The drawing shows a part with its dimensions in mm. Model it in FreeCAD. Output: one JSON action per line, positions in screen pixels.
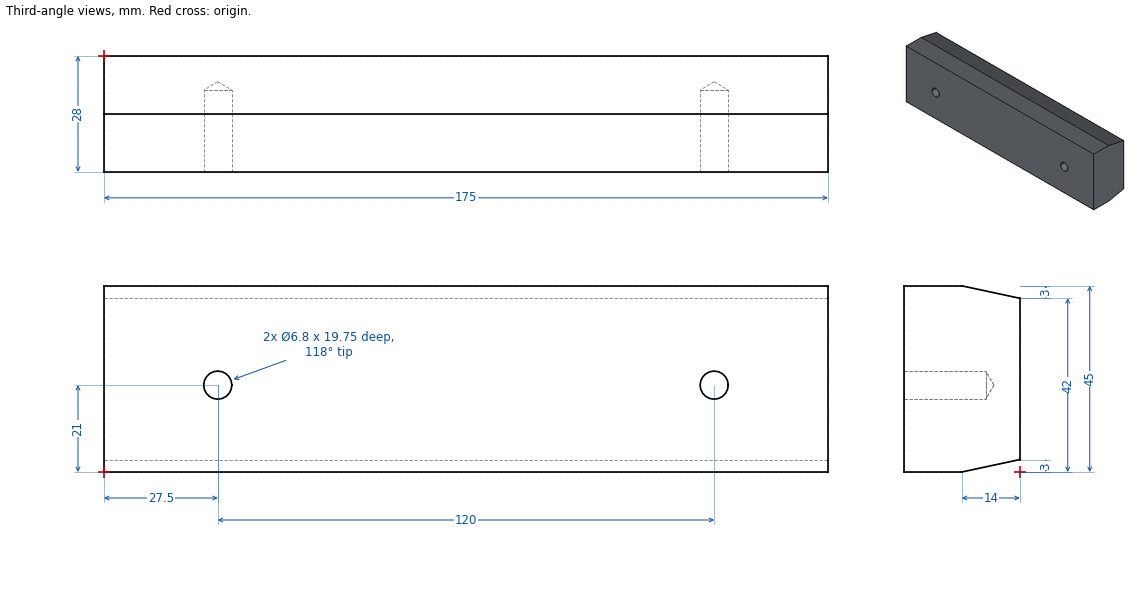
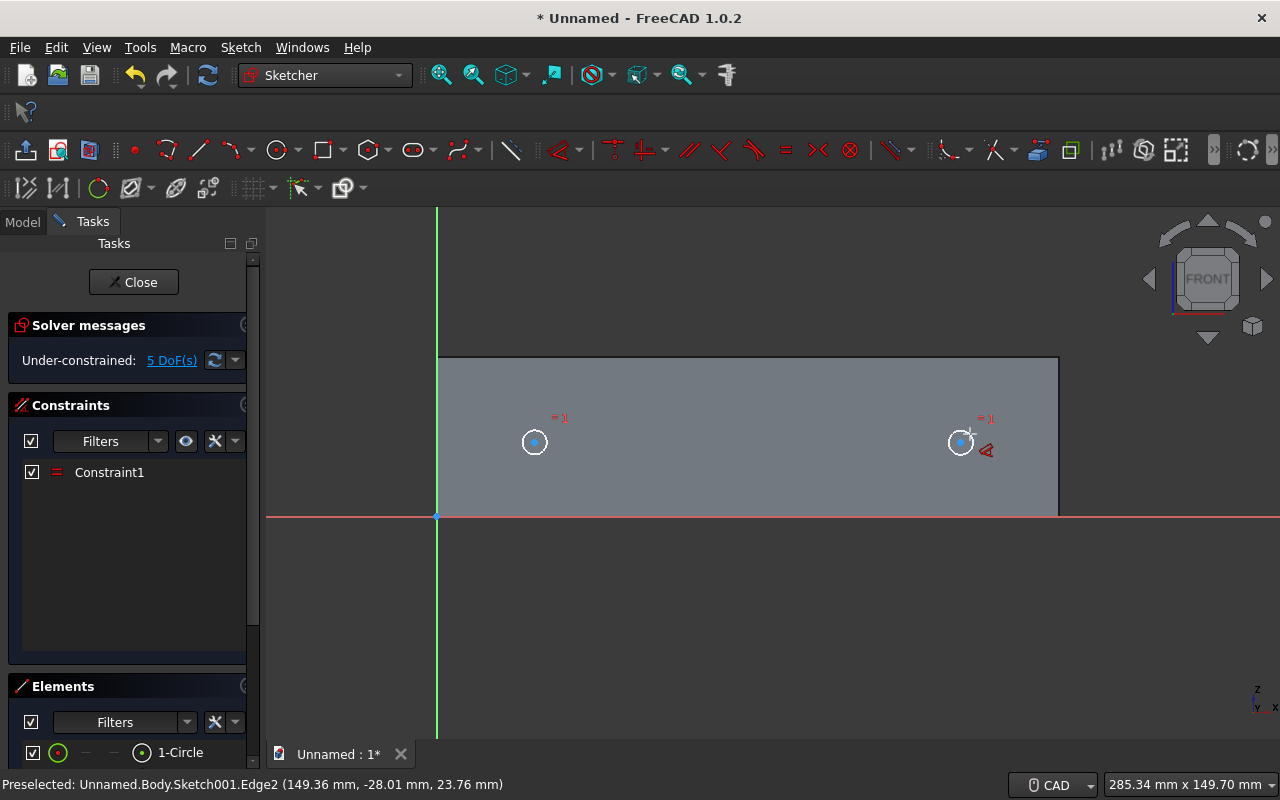
{"action": "scroll", "coordinate": [543, 434], "scroll_direction": "up", "scroll_amount": 3}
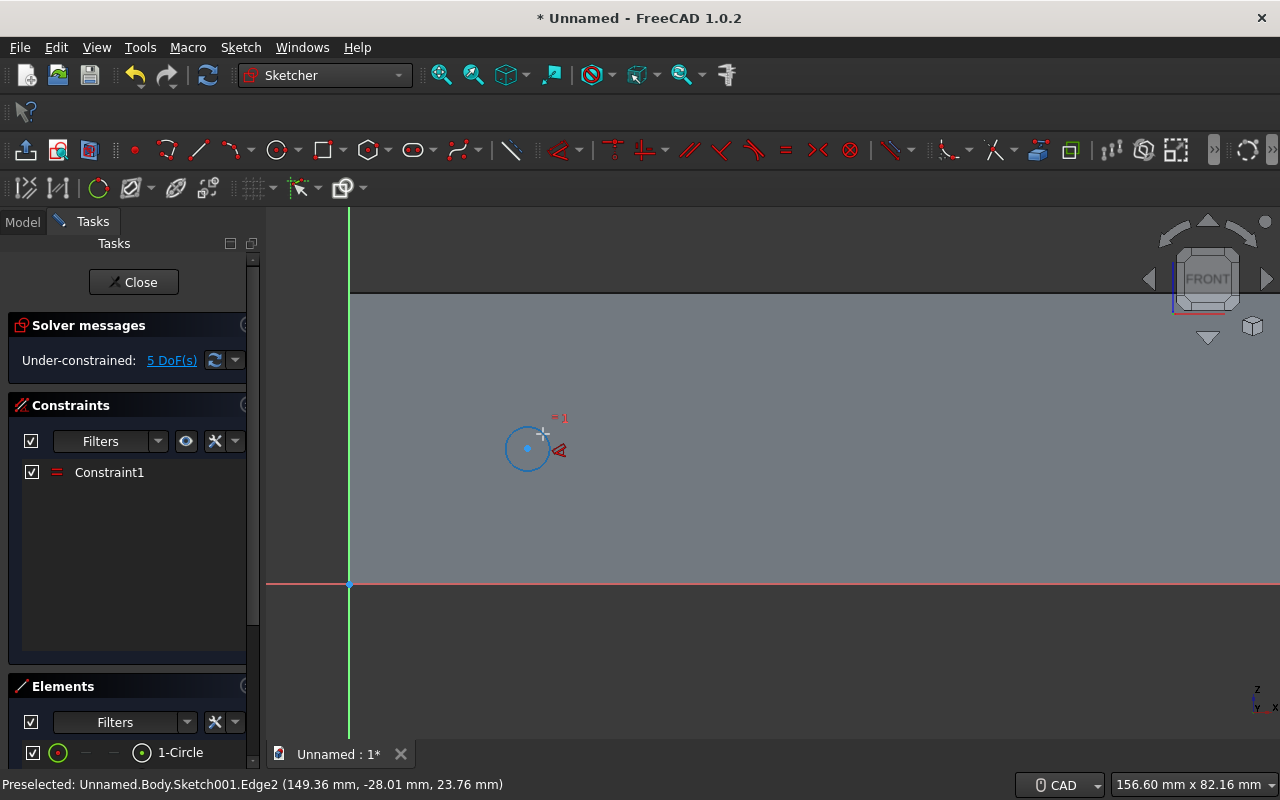
{"action": "left_click", "coordinate": [543, 433]}
{"action": "left_click", "coordinate": [565, 410]}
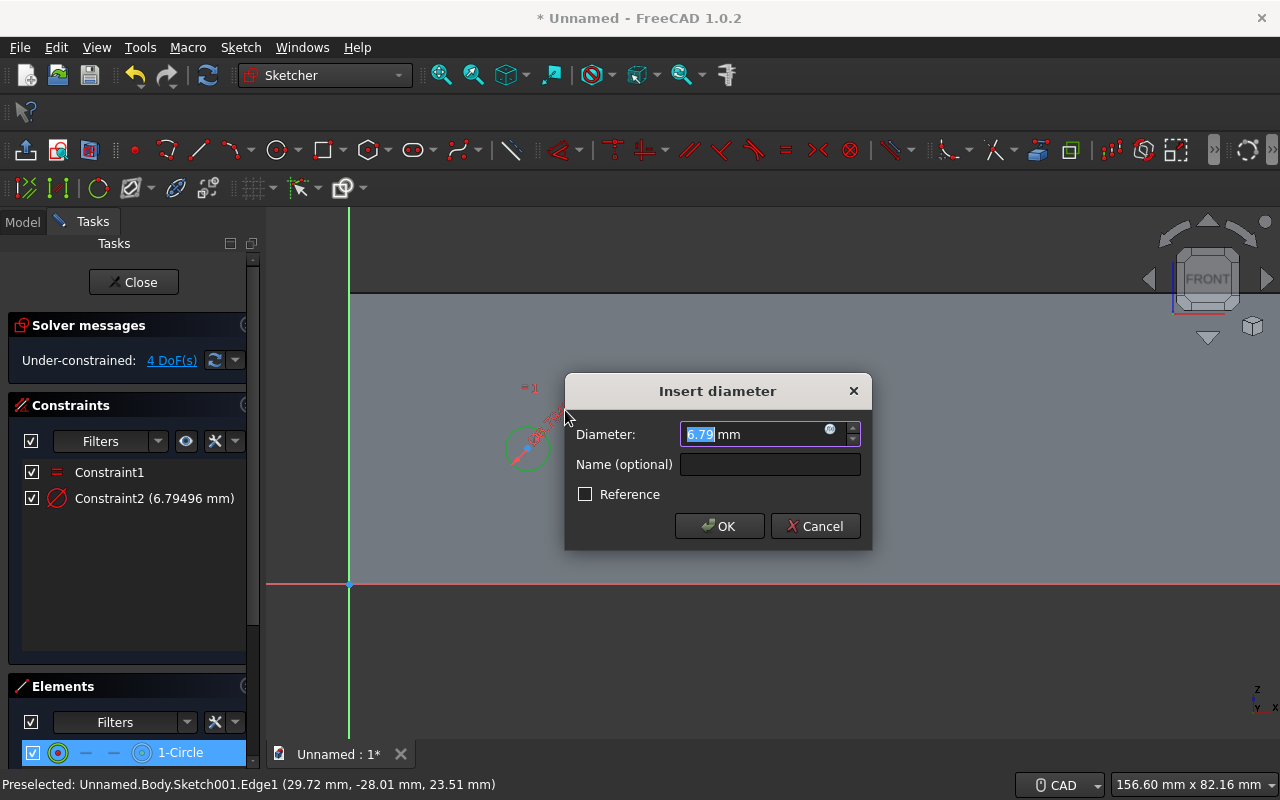
{"action": "type", "text": "6.8"}
{"action": "key", "text": "Return"}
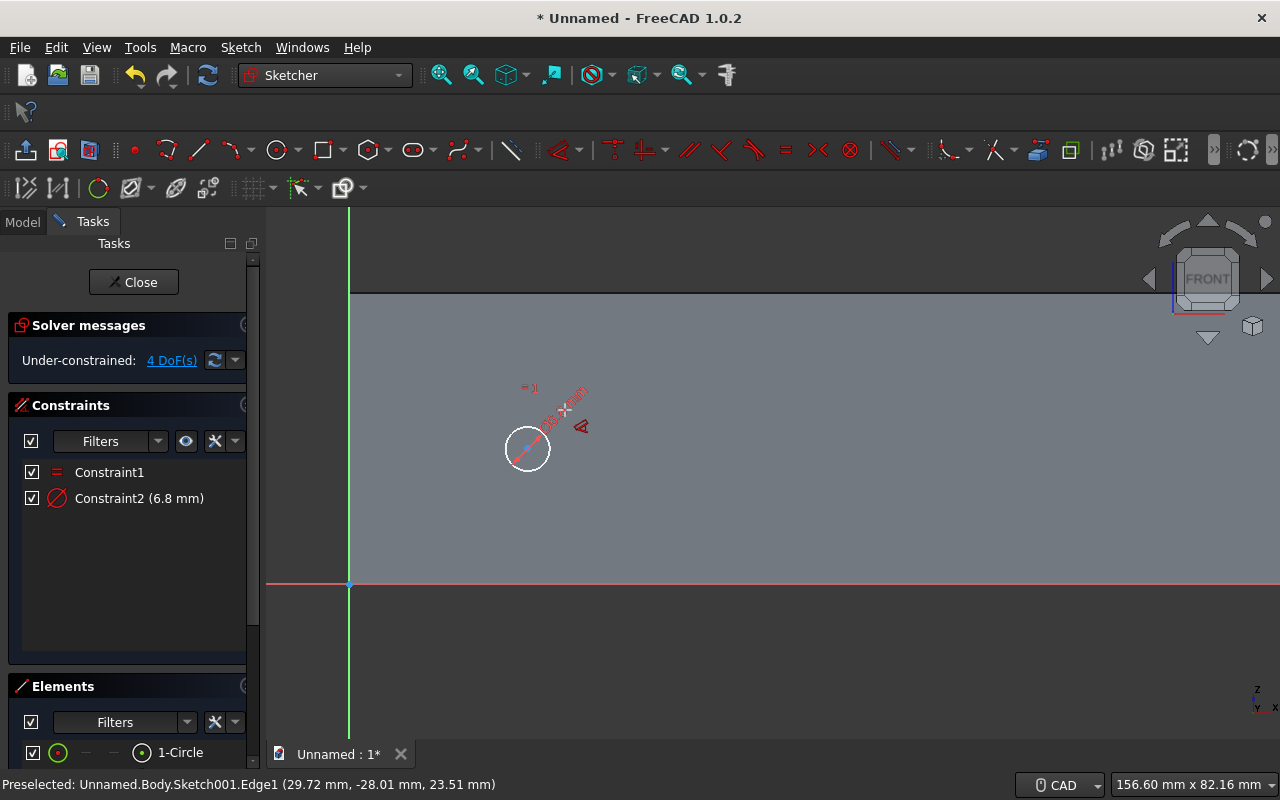
{"action": "left_click", "coordinate": [528, 449]}
{"action": "left_click", "coordinate": [315, 517]}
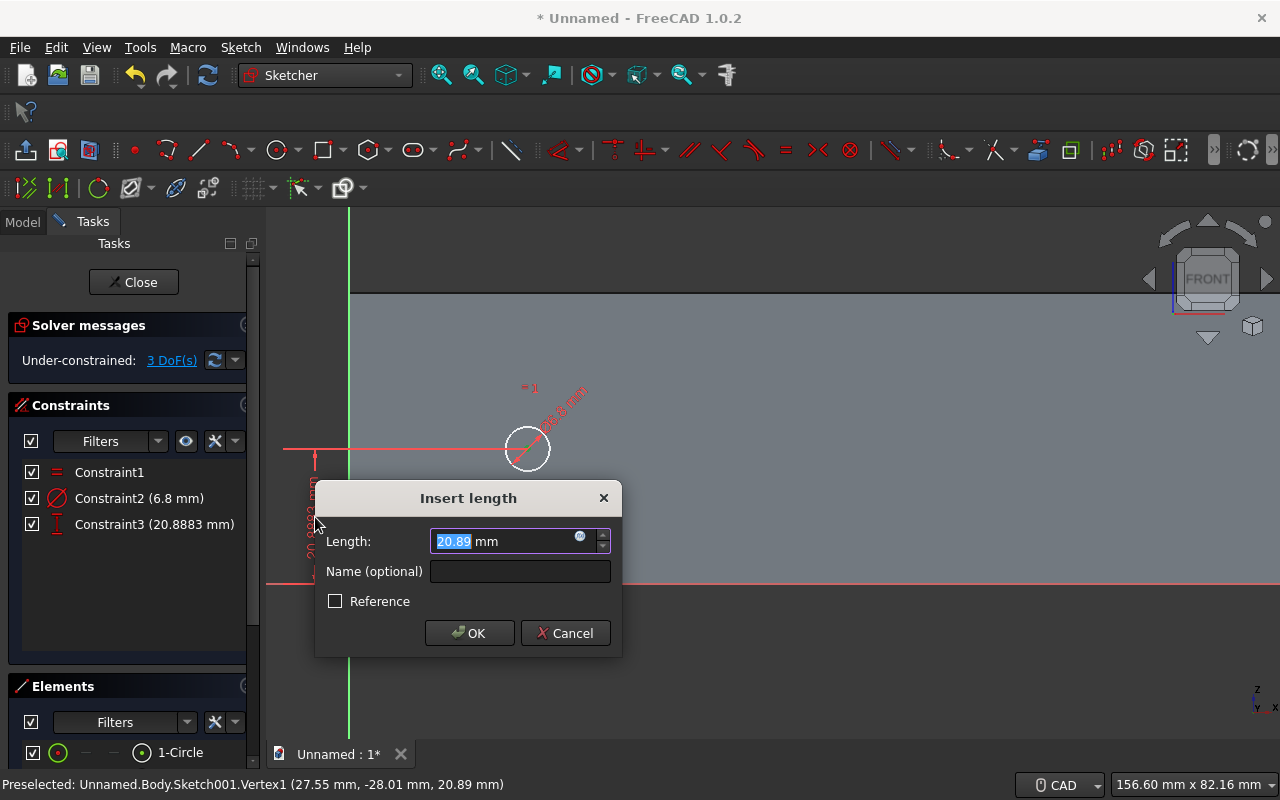
{"action": "type", "text": "21"}
{"action": "key", "text": "Return"}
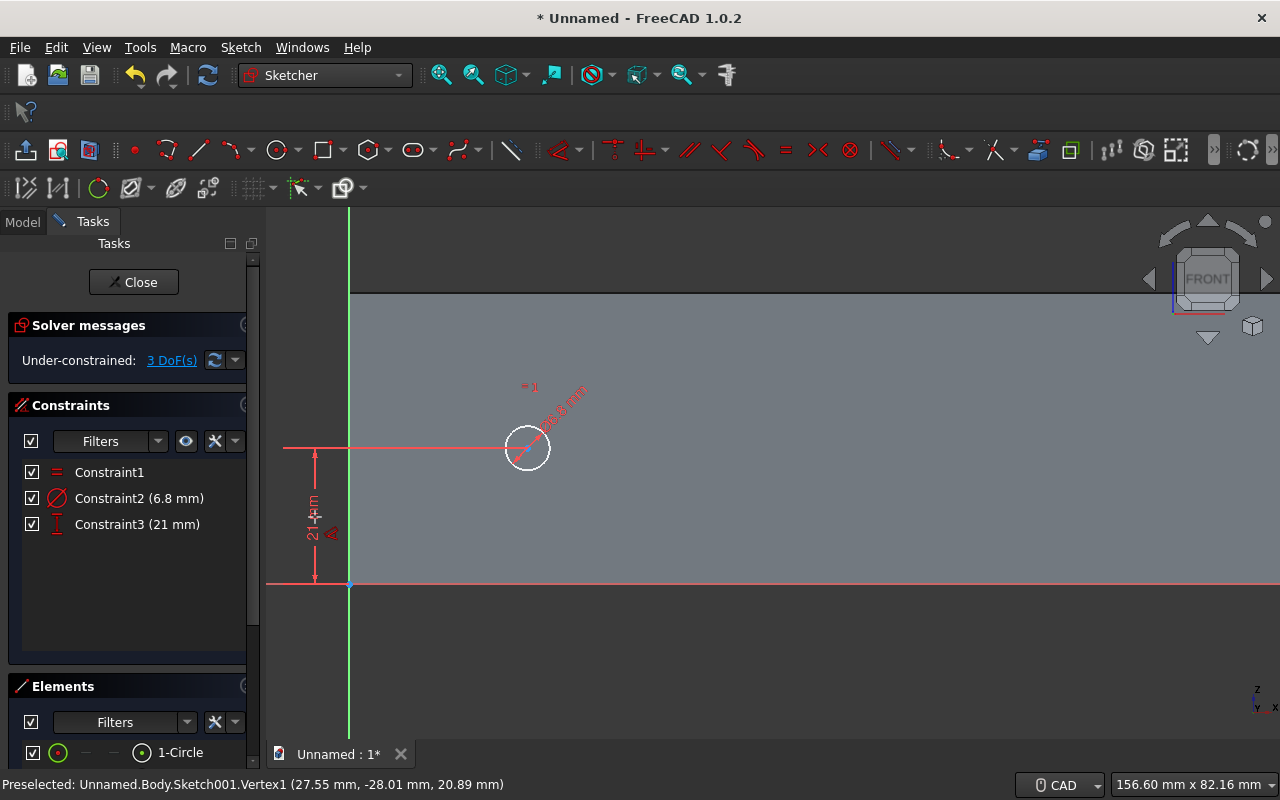
{"action": "scroll", "coordinate": [542, 434], "scroll_direction": "down", "scroll_amount": 3}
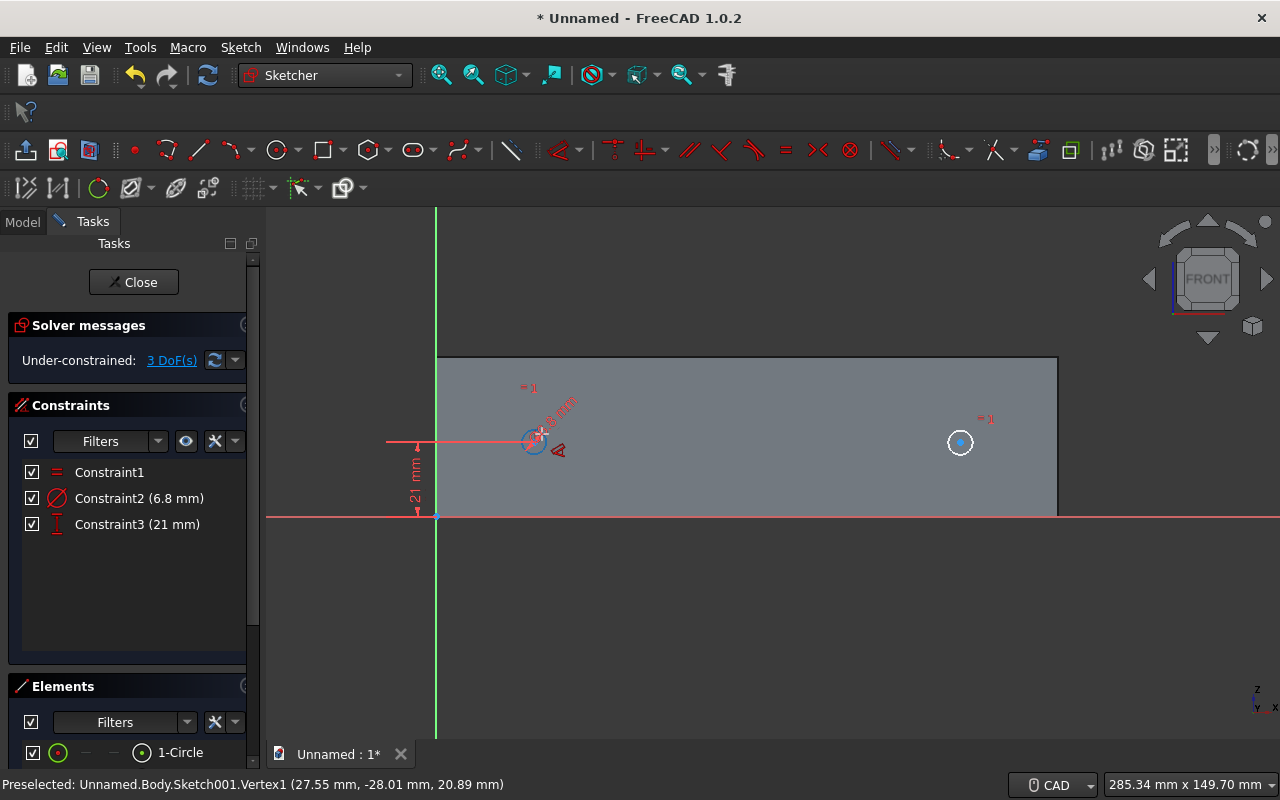
{"action": "left_click", "coordinate": [960, 443]}
{"action": "left_click", "coordinate": [402, 454]}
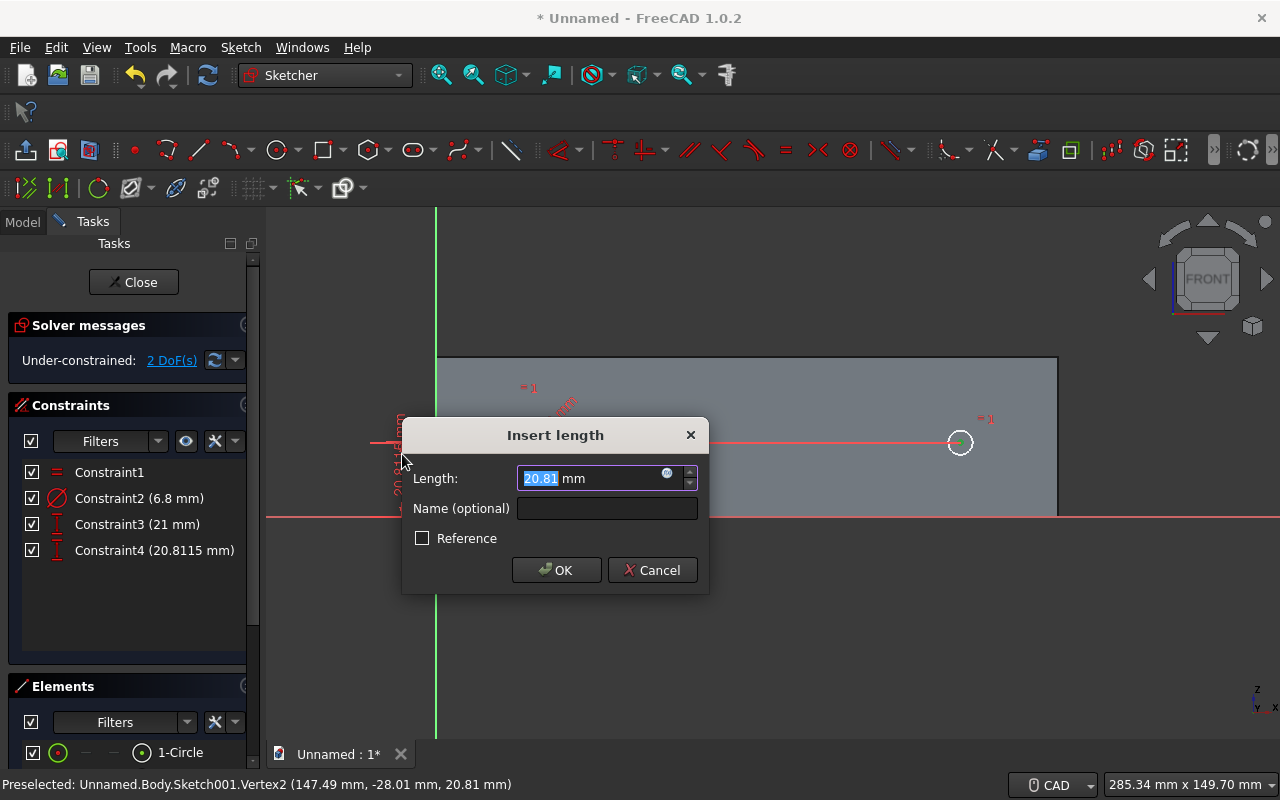
{"action": "type", "text": "21"}
{"action": "key", "text": "Return"}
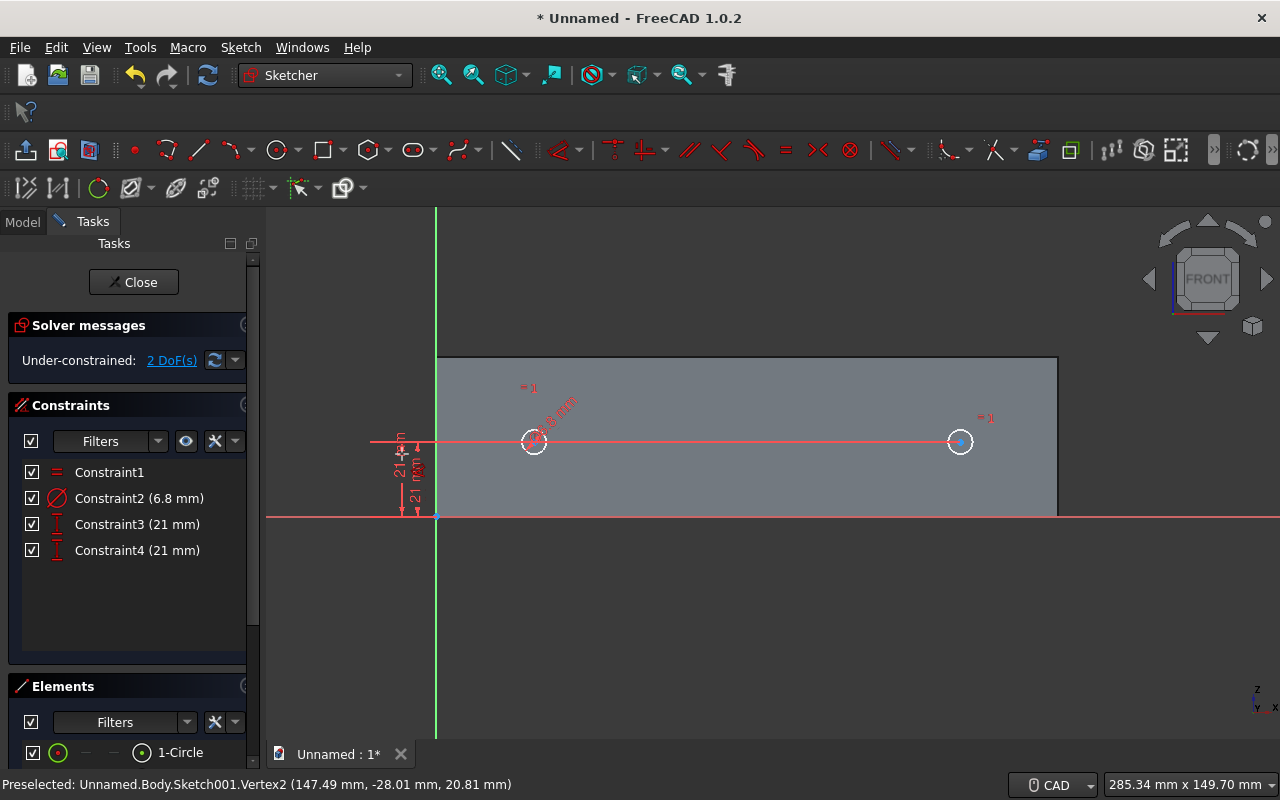
{"action": "left_click", "coordinate": [534, 442]}
{"action": "left_click", "coordinate": [485, 551]}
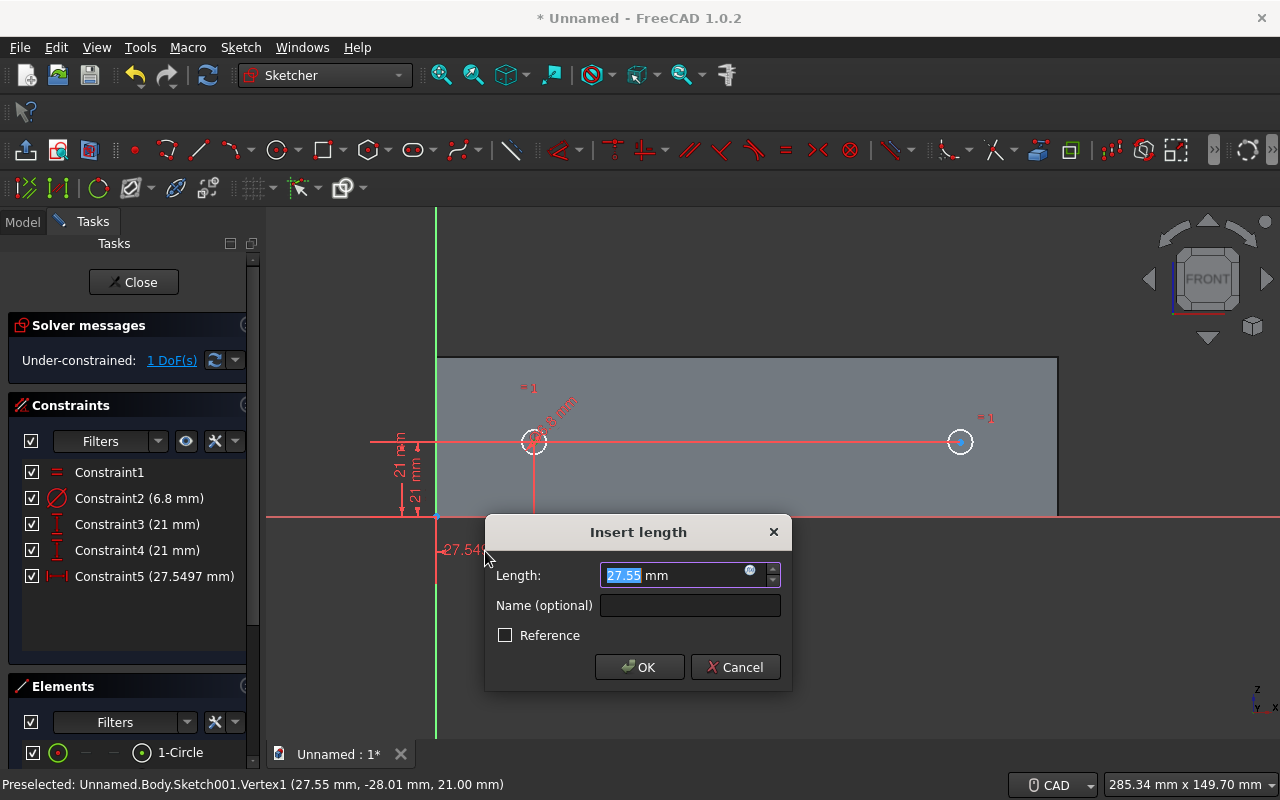
{"action": "type", "text": "27.5"}
{"action": "key", "text": "Return"}